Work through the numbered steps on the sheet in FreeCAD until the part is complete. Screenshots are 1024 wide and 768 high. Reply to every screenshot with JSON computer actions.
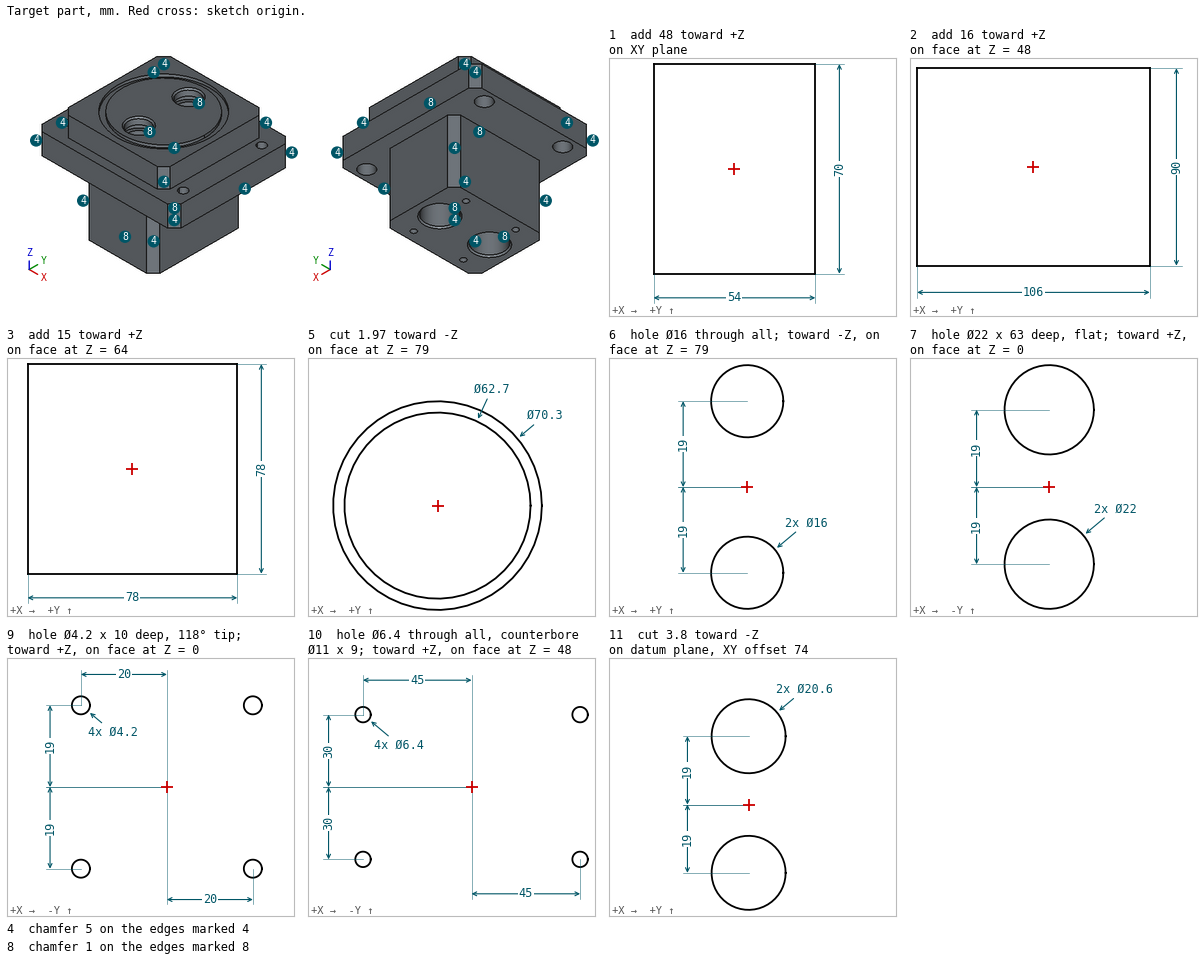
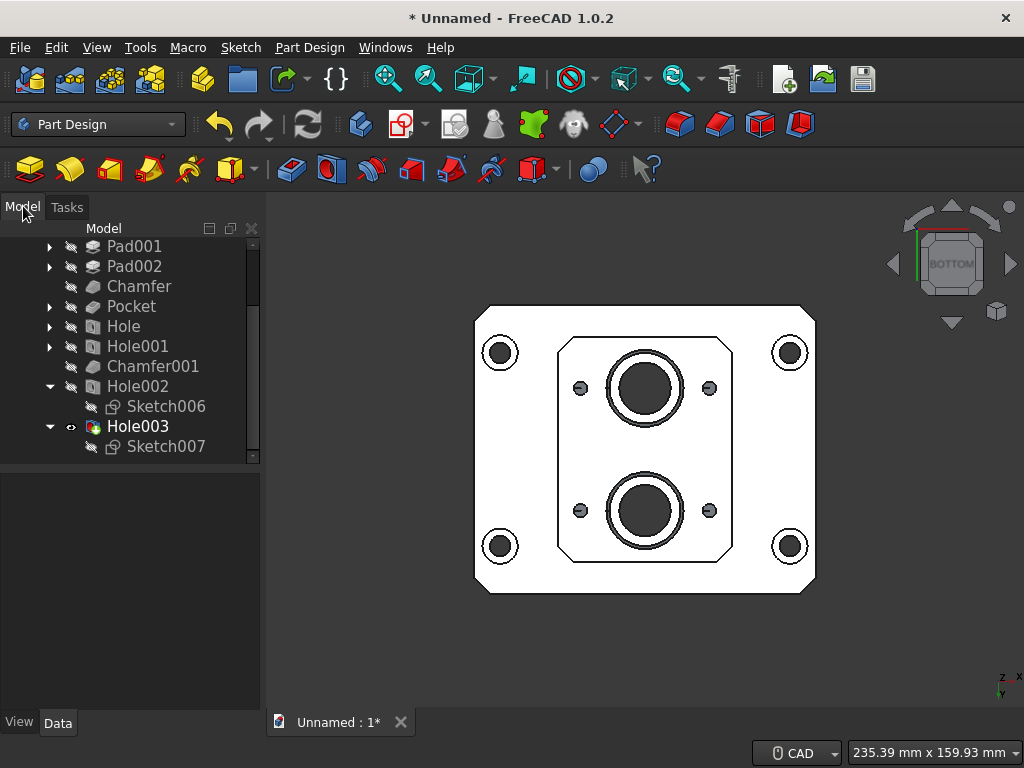
{"action": "scroll", "coordinate": [140, 342], "scroll_direction": "down", "scroll_amount": 3}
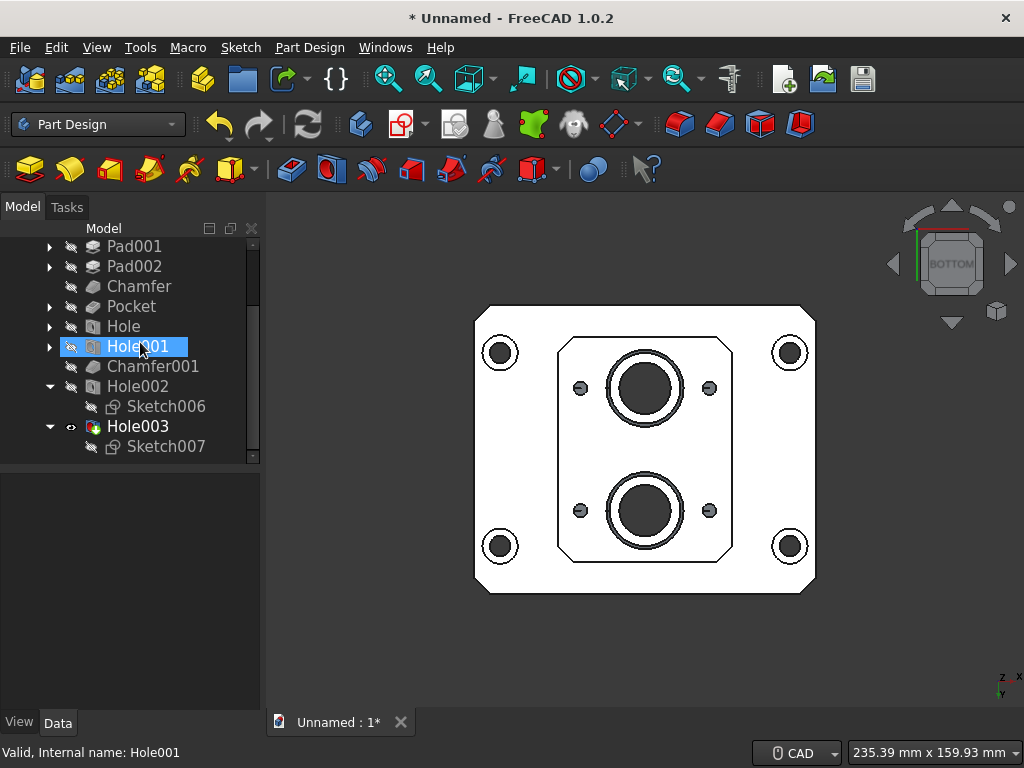
{"action": "scroll", "coordinate": [140, 342], "scroll_direction": "up", "scroll_amount": 15}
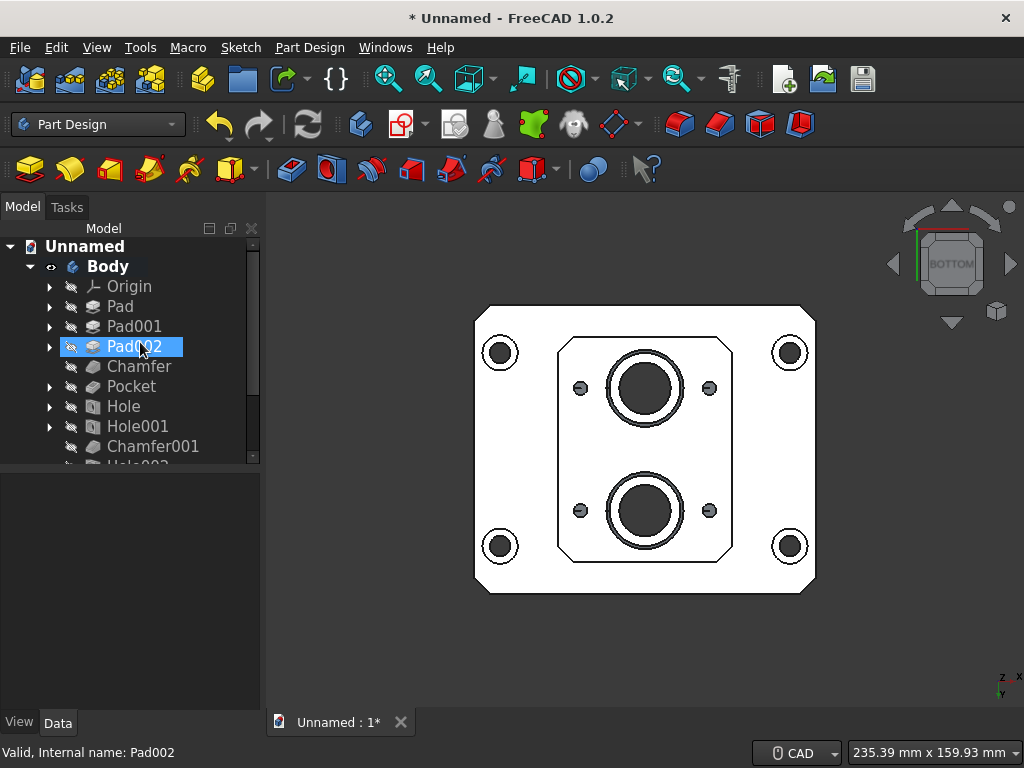
{"action": "left_click", "coordinate": [50, 287]}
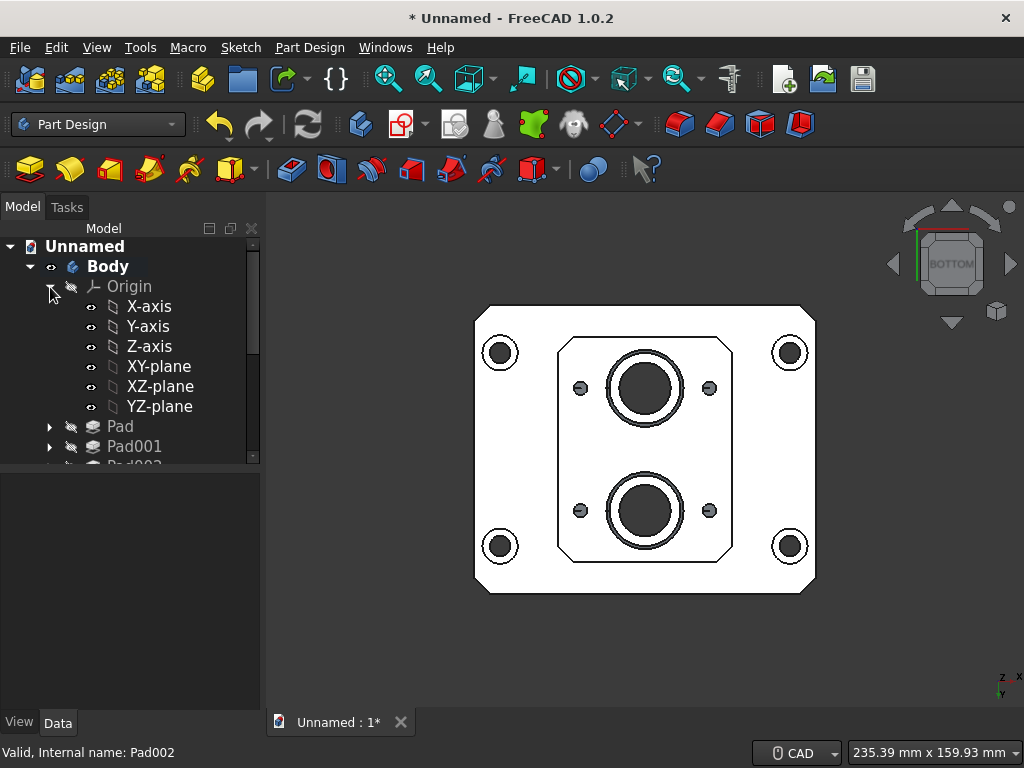
{"action": "left_click", "coordinate": [136, 367]}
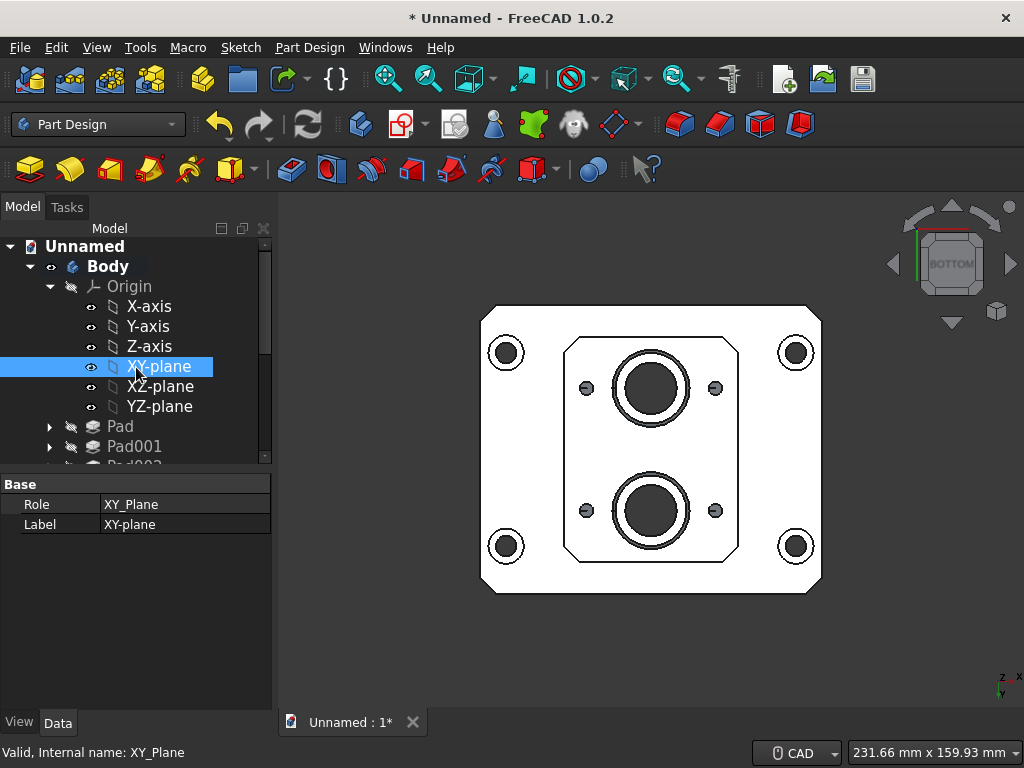
{"action": "left_click", "coordinate": [614, 124]}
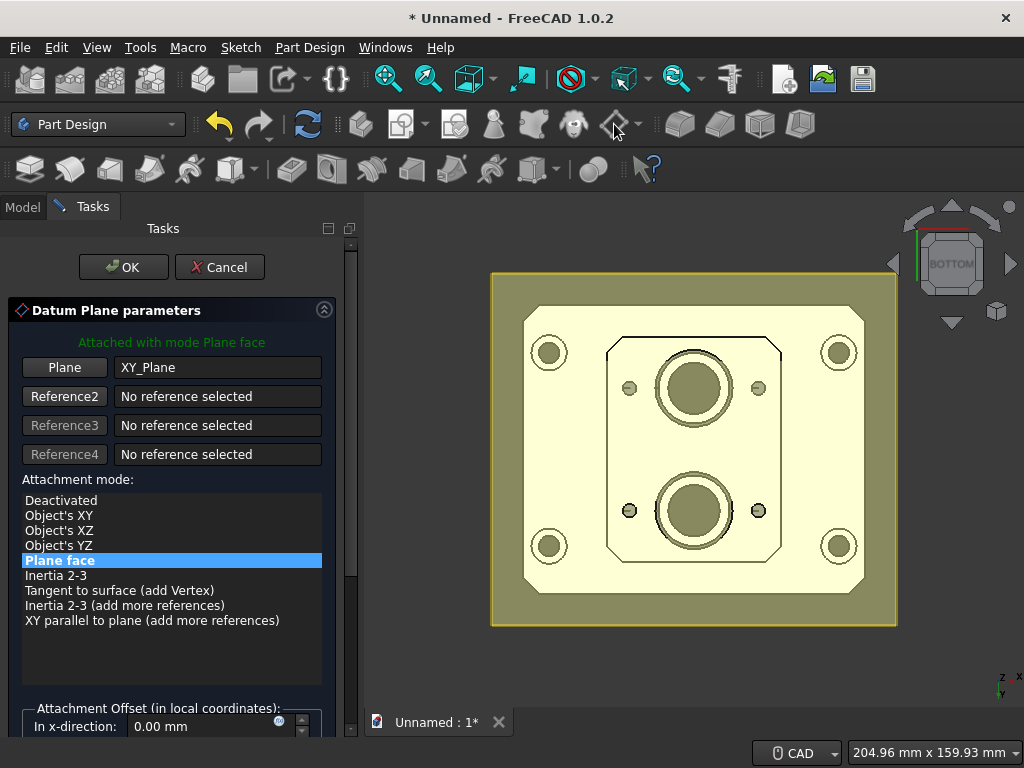
{"action": "scroll", "coordinate": [351, 487], "scroll_direction": "down", "scroll_amount": 3}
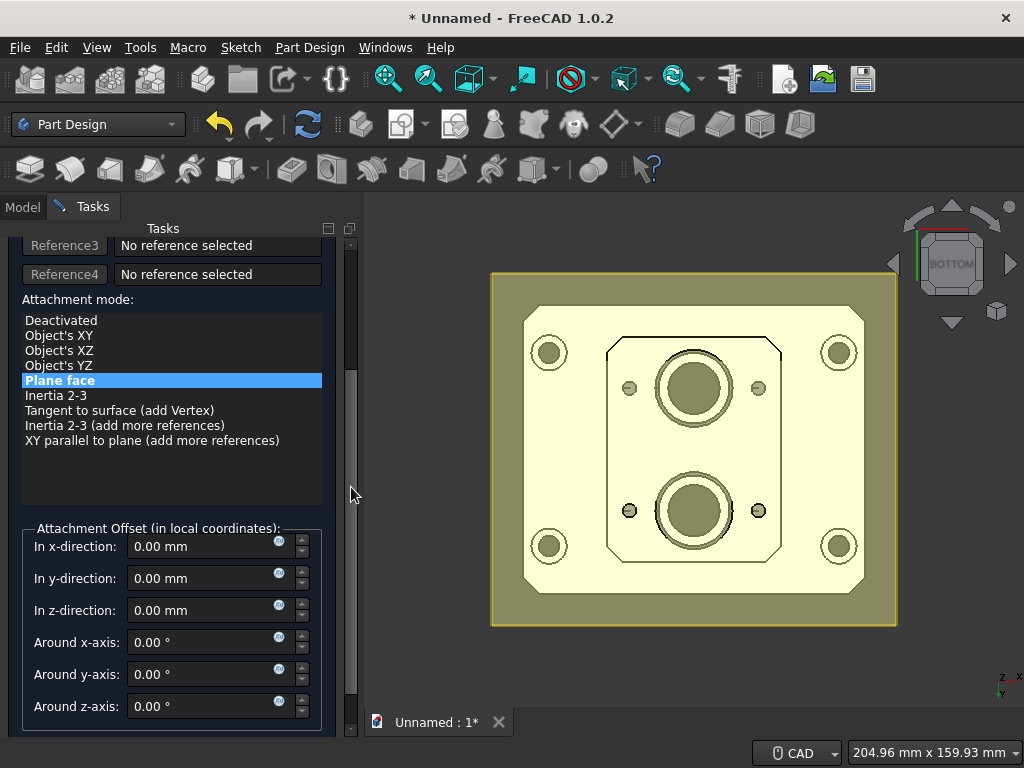
{"action": "triple_click", "coordinate": [210, 610]}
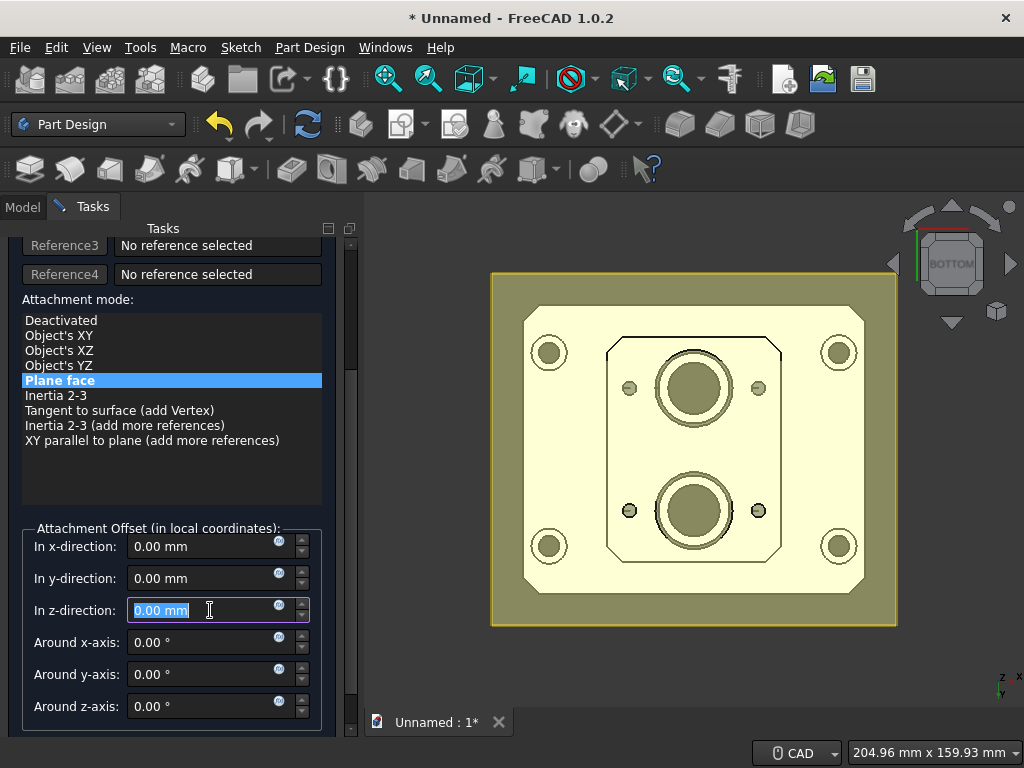
{"action": "type", "text": "74"}
{"action": "key", "text": "Tab"}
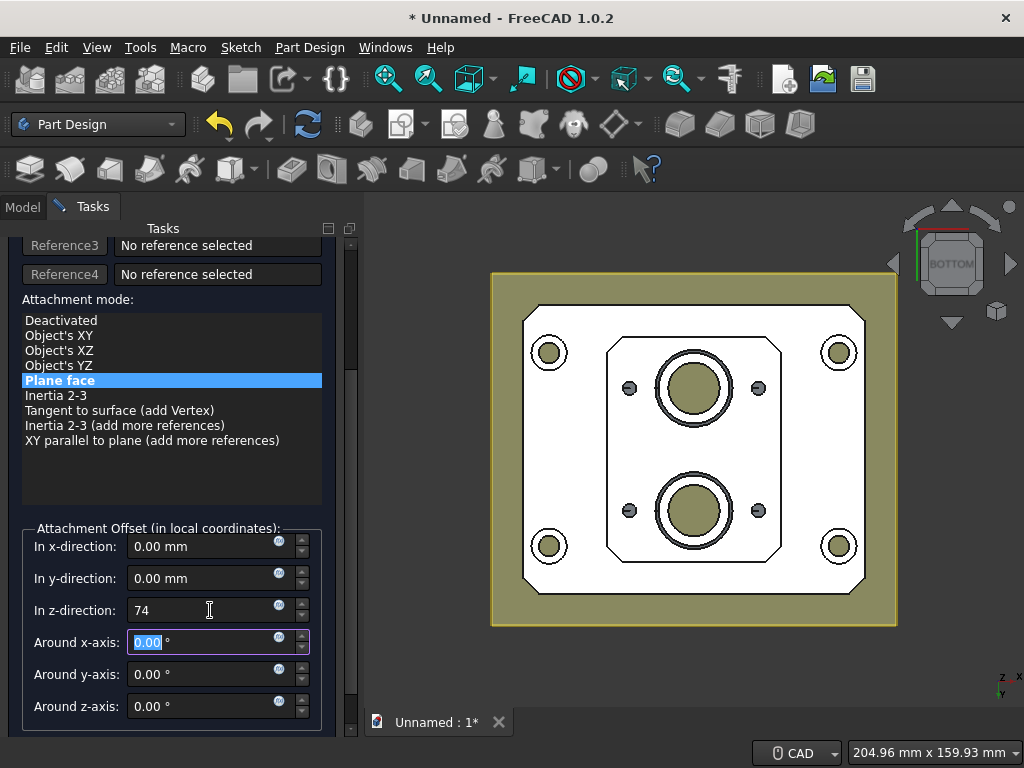
{"action": "scroll", "coordinate": [351, 487], "scroll_direction": "up", "scroll_amount": 4}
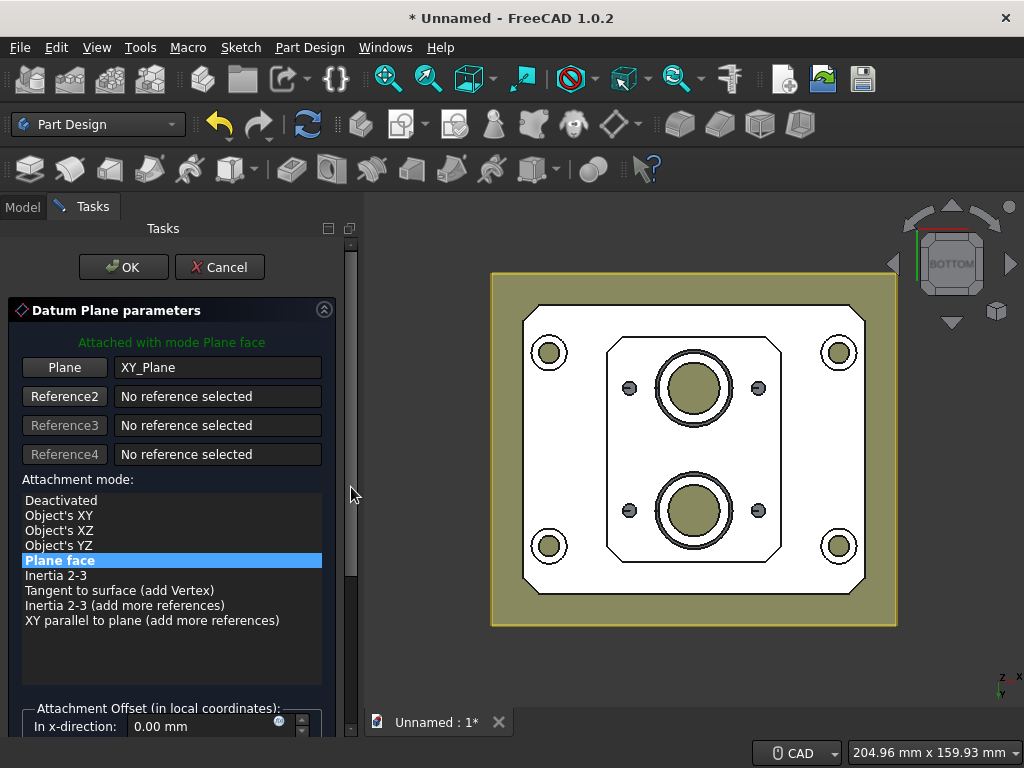
{"action": "left_click", "coordinate": [124, 267]}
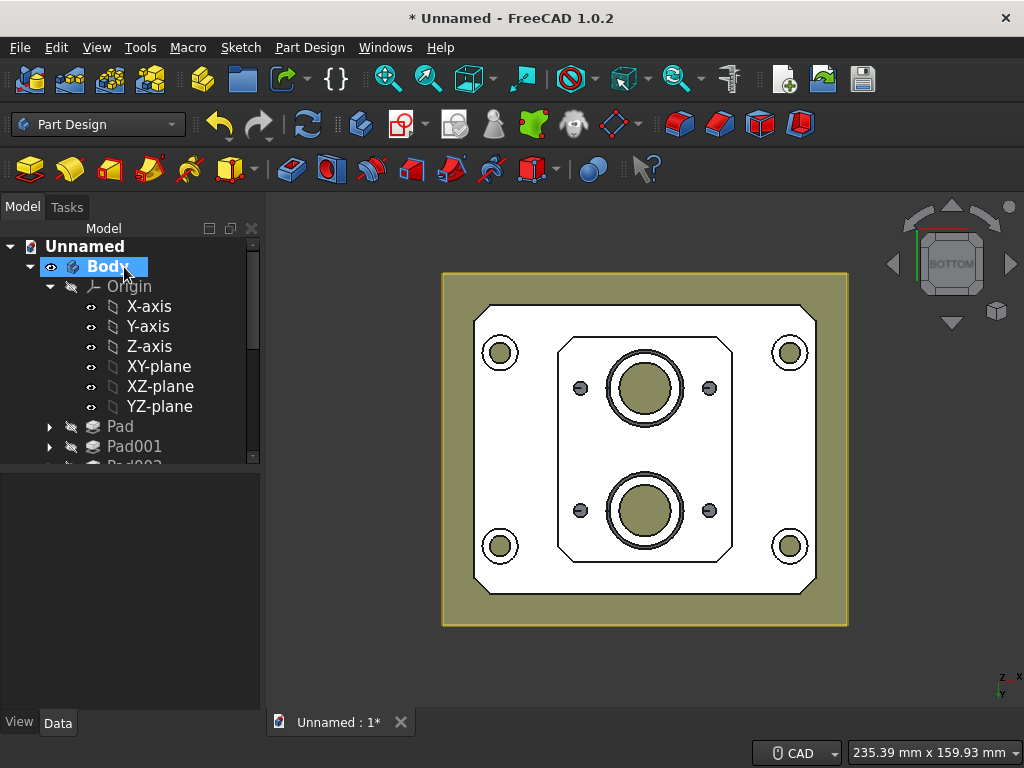
{"action": "scroll", "coordinate": [100, 342], "scroll_direction": "down", "scroll_amount": 3}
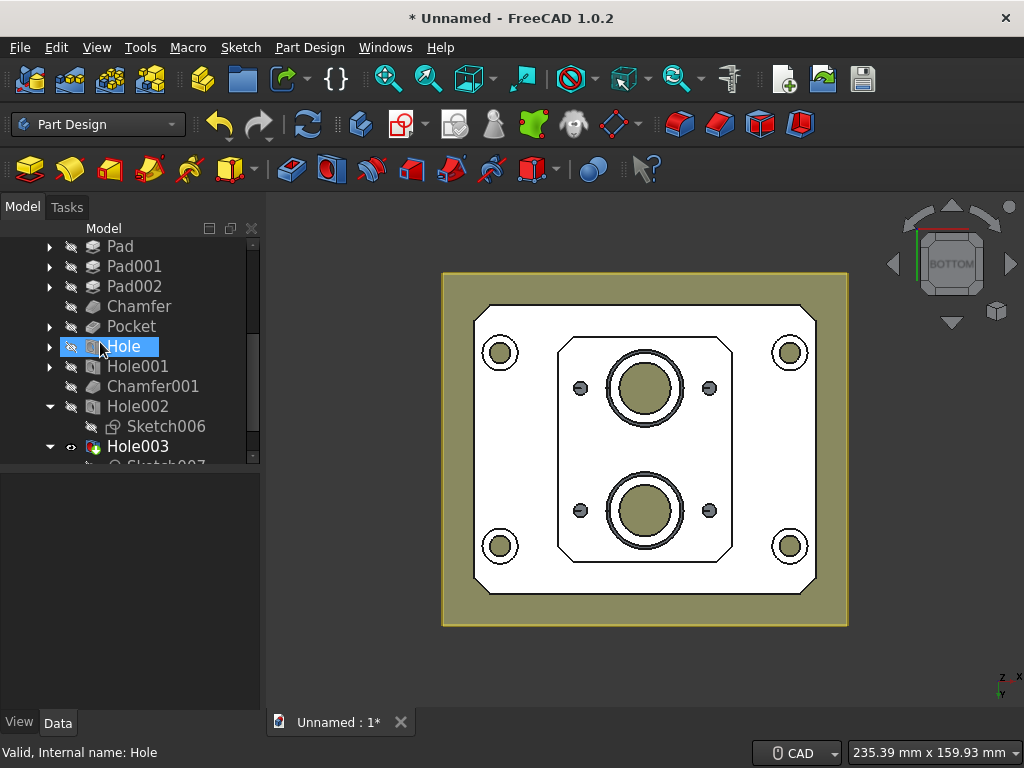
{"action": "scroll", "coordinate": [140, 342], "scroll_direction": "up", "scroll_amount": 15}